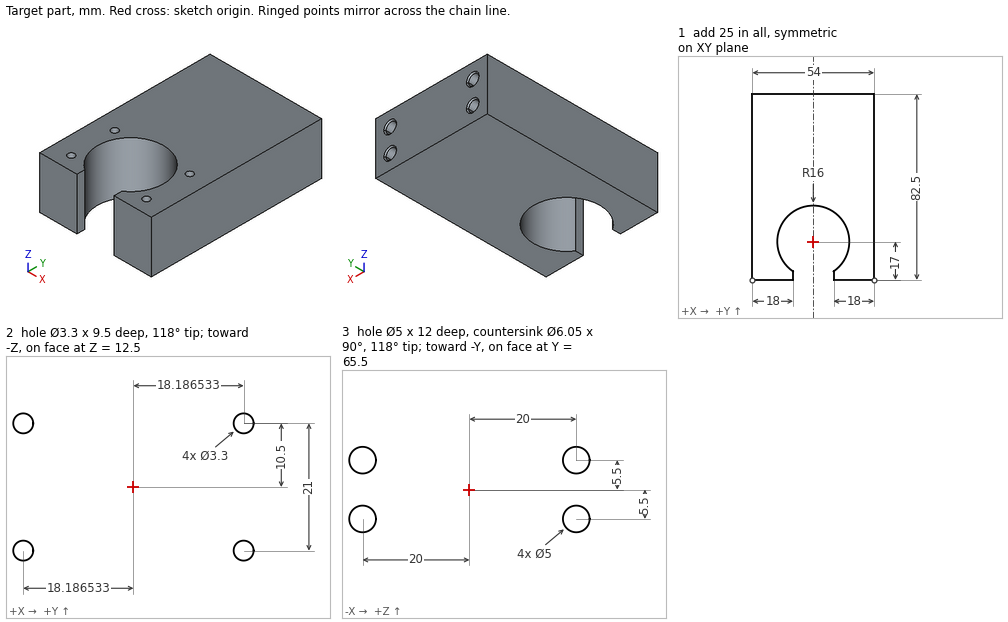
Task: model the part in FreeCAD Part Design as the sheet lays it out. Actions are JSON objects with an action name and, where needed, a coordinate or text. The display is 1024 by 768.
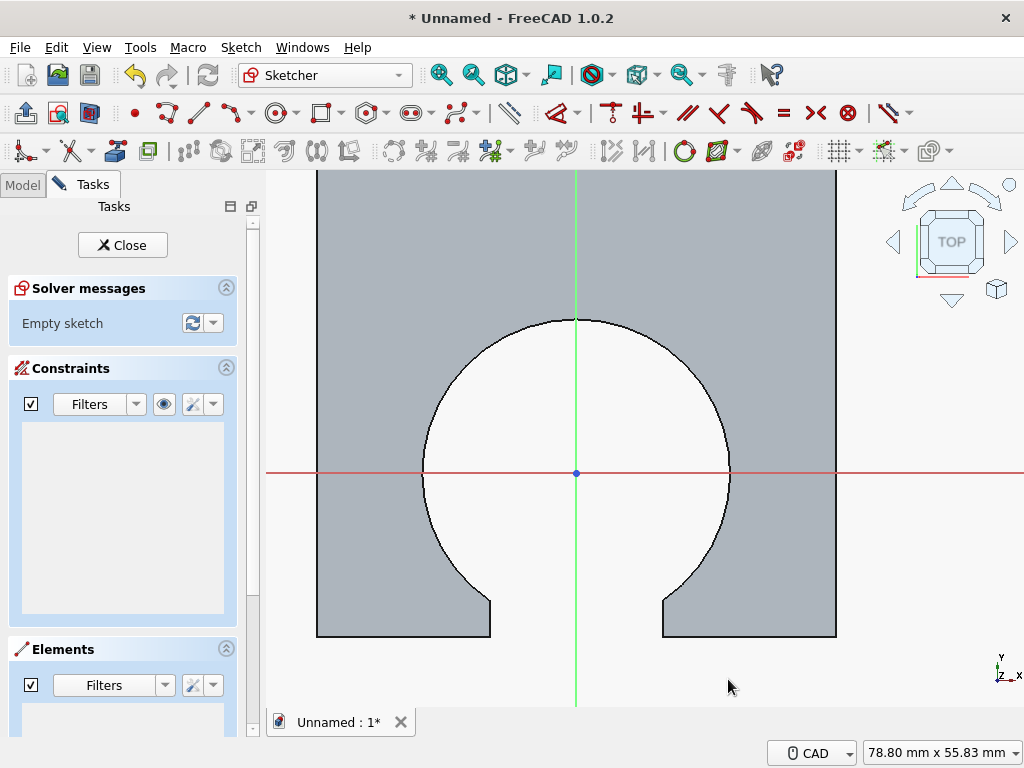
{"action": "left_click", "coordinate": [276, 114]}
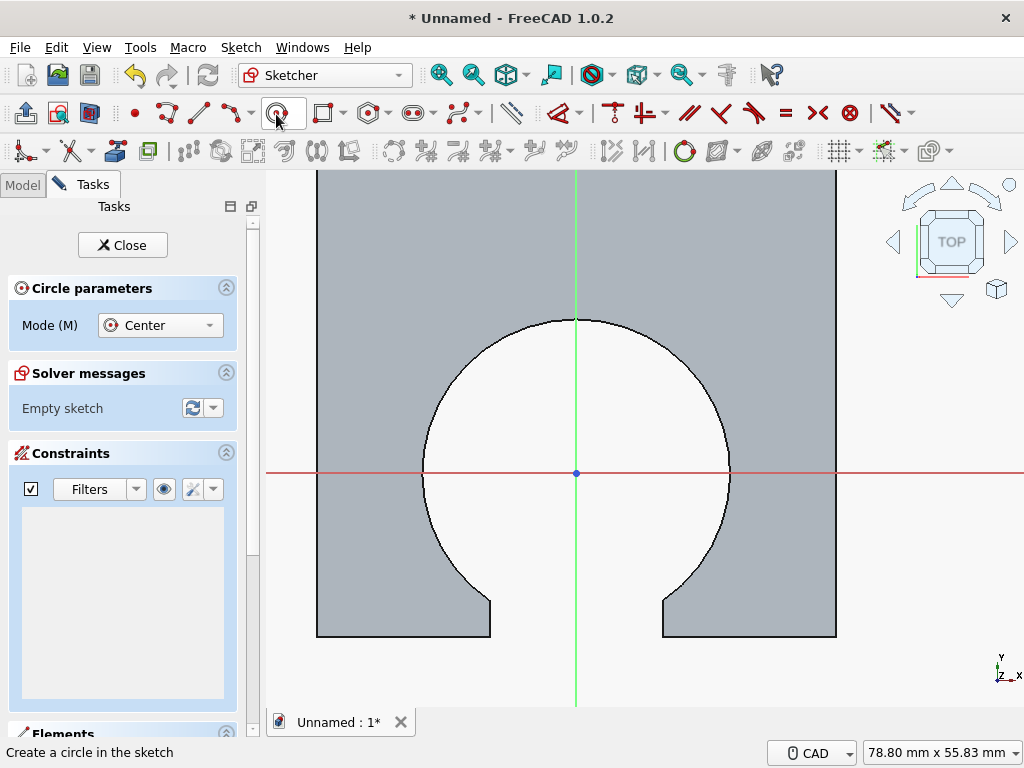
{"action": "scroll", "coordinate": [751, 372], "scroll_direction": "up", "scroll_amount": 2}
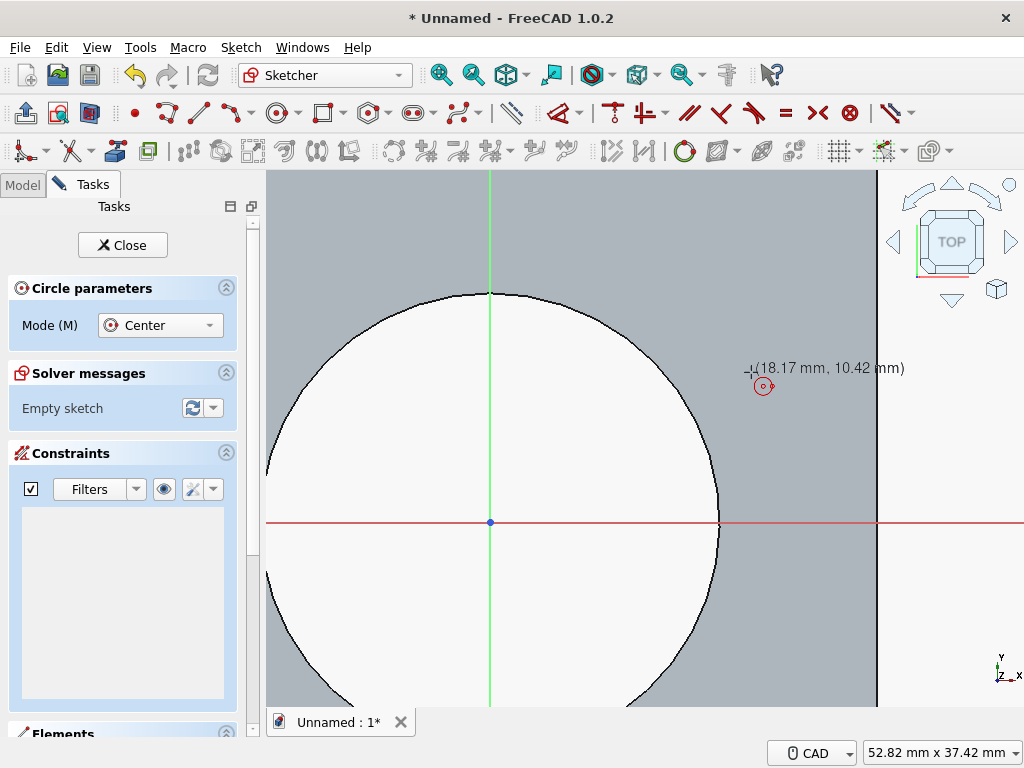
{"action": "left_click", "coordinate": [751, 372]}
{"action": "left_click", "coordinate": [768, 355]}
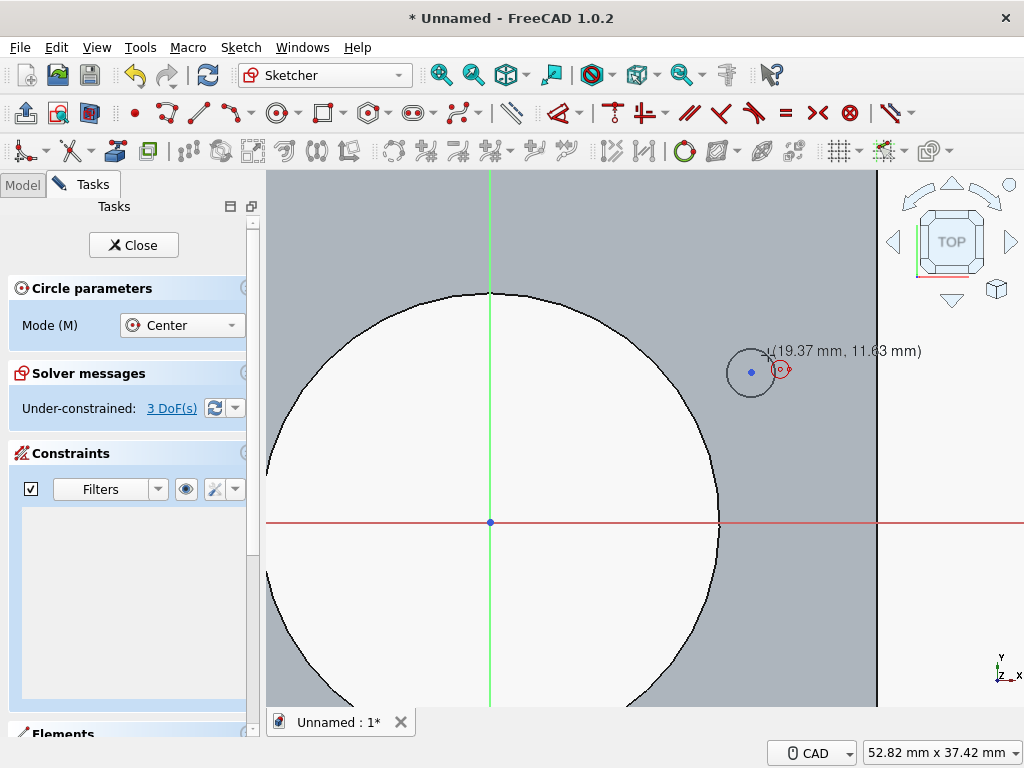
{"action": "left_click", "coordinate": [751, 674]}
{"action": "left_click", "coordinate": [768, 657]}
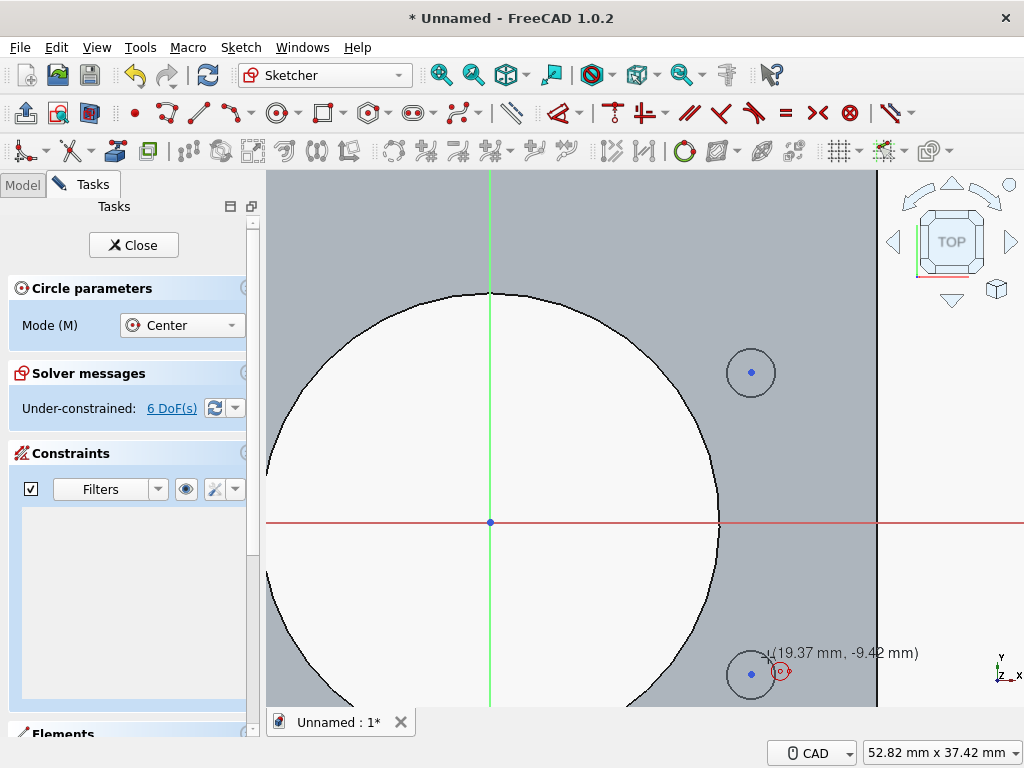
{"action": "scroll", "coordinate": [752, 267], "scroll_direction": "down", "scroll_amount": 2}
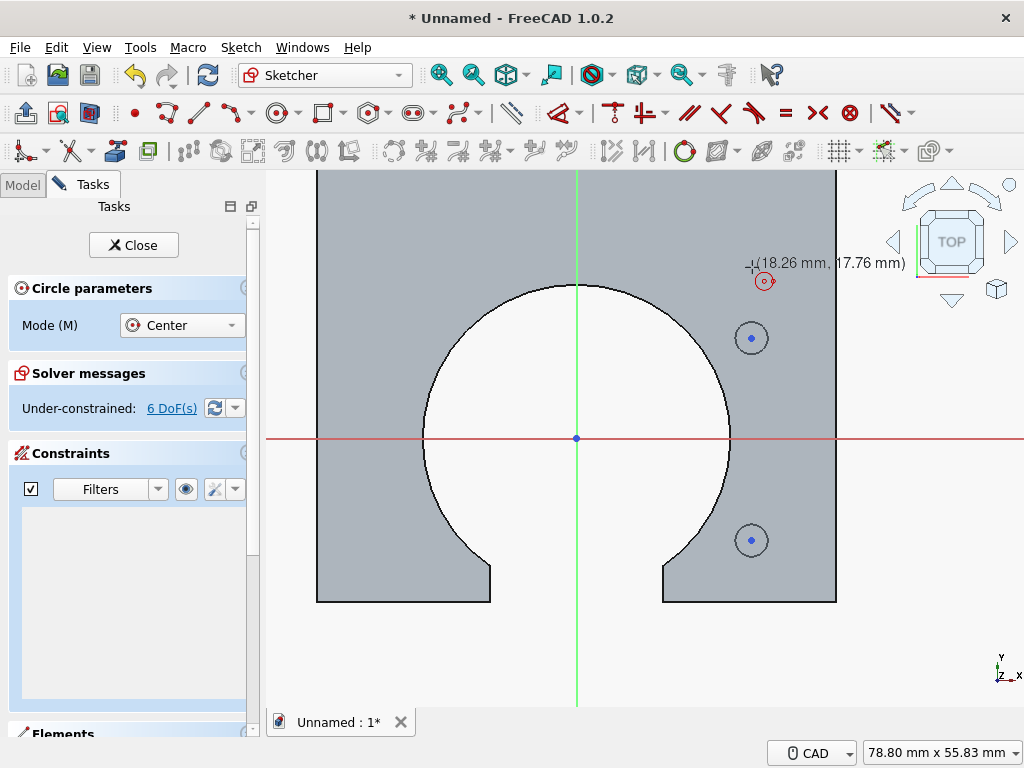
{"action": "scroll", "coordinate": [402, 540], "scroll_direction": "up", "scroll_amount": 2}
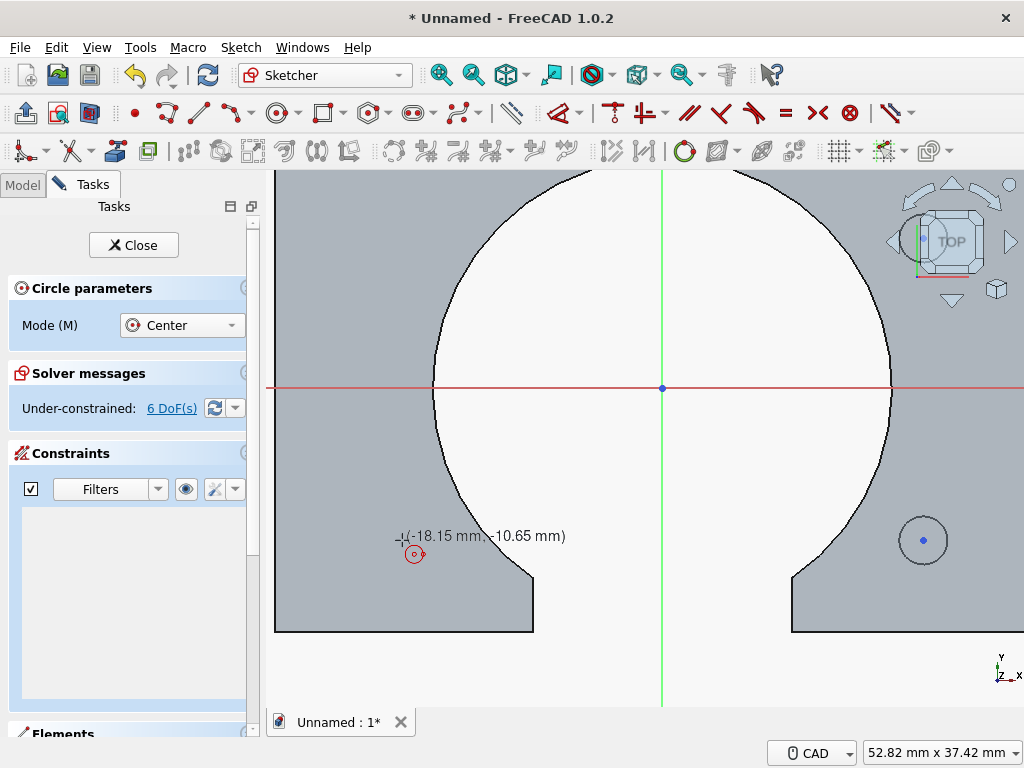
{"action": "left_click", "coordinate": [401, 539]}
{"action": "left_click", "coordinate": [418, 522]}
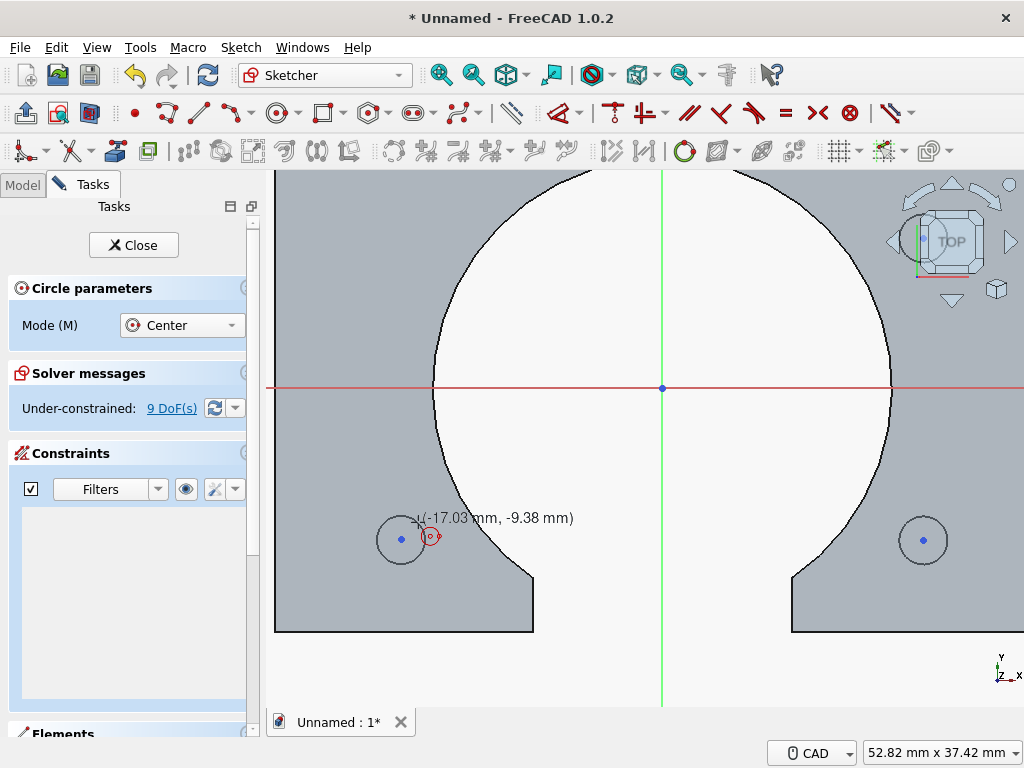
{"action": "left_click", "coordinate": [401, 238]}
{"action": "left_click", "coordinate": [418, 221]}
{"action": "key", "text": "Escape"}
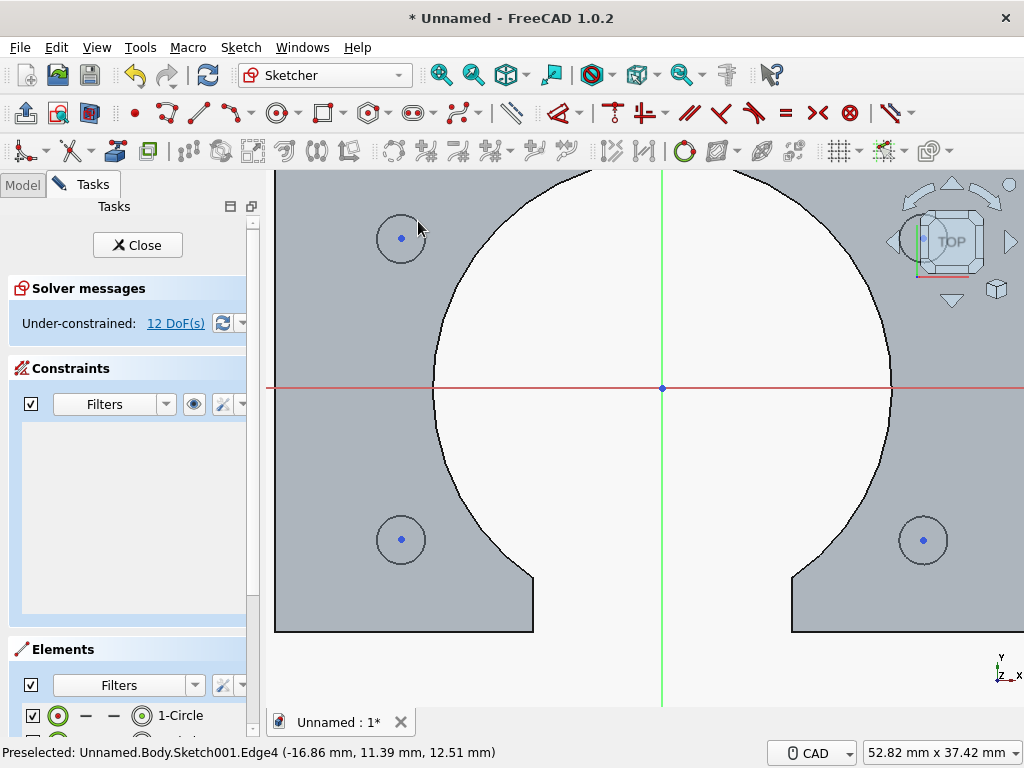
{"action": "scroll", "coordinate": [402, 540], "scroll_direction": "down", "scroll_amount": 2}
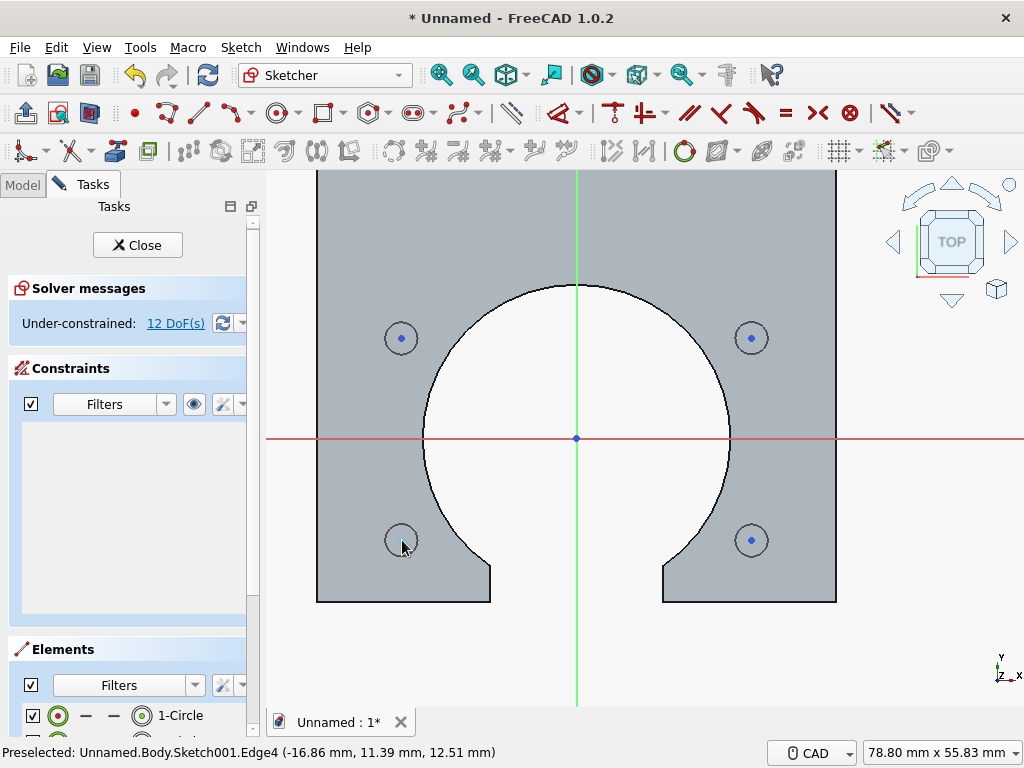
{"action": "left_click", "coordinate": [763, 327]}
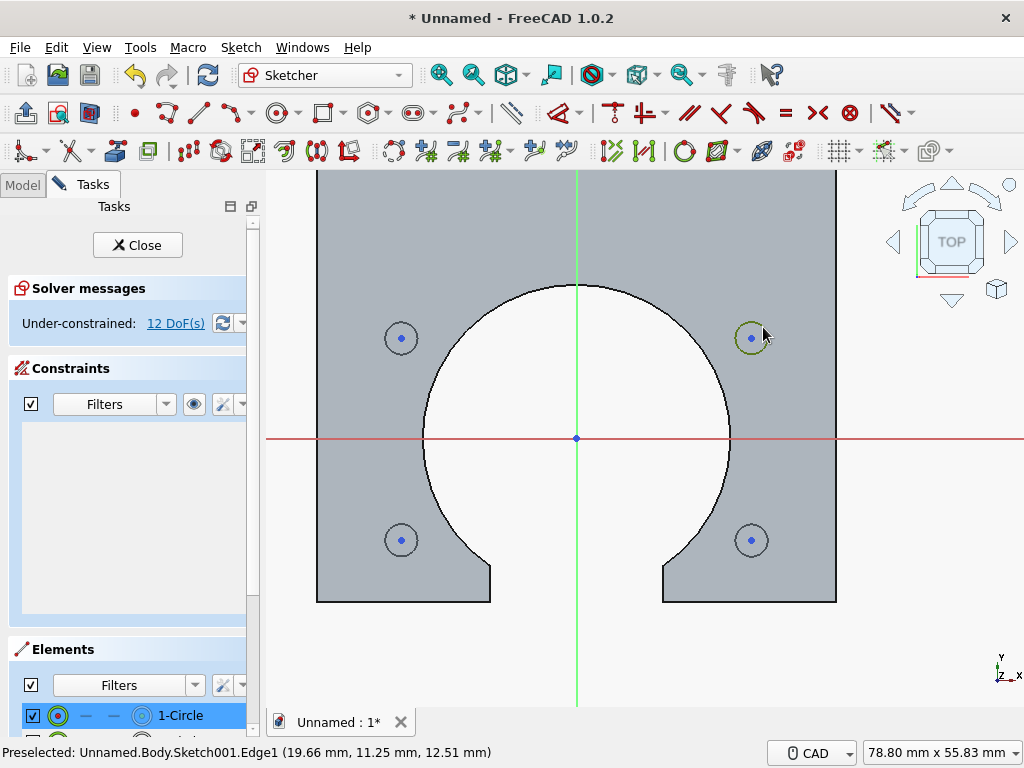
{"action": "left_click", "coordinate": [763, 529]}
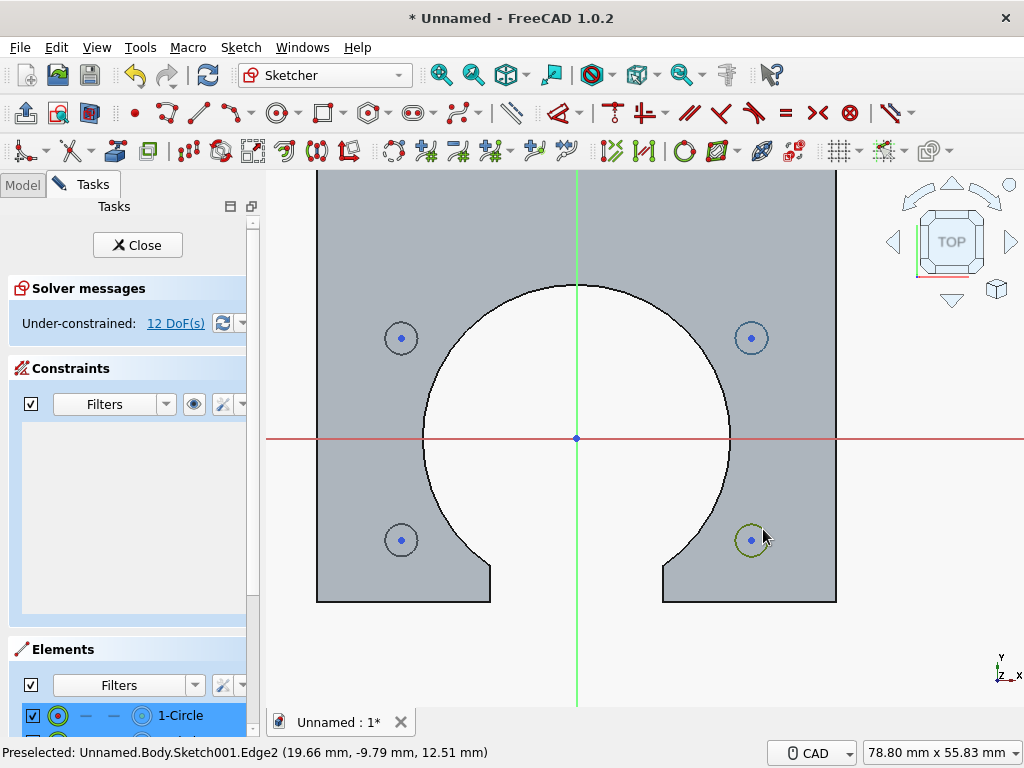
{"action": "left_click", "coordinate": [413, 529]}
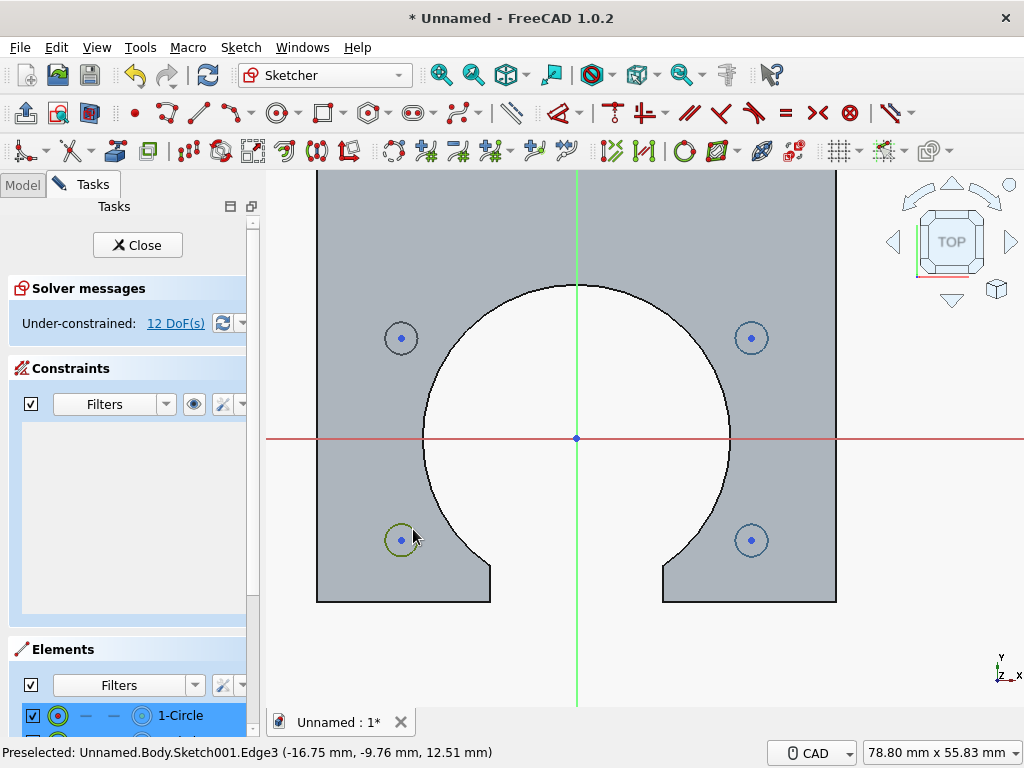
{"action": "left_click", "coordinate": [413, 327]}